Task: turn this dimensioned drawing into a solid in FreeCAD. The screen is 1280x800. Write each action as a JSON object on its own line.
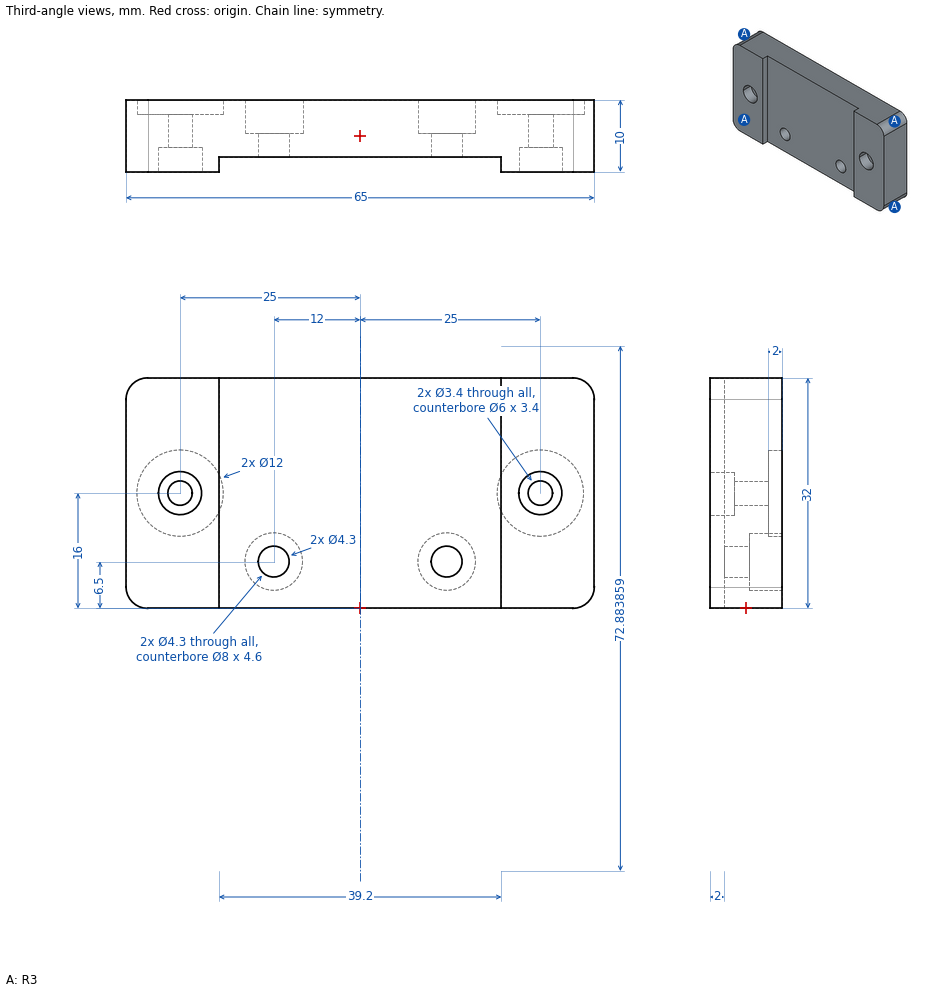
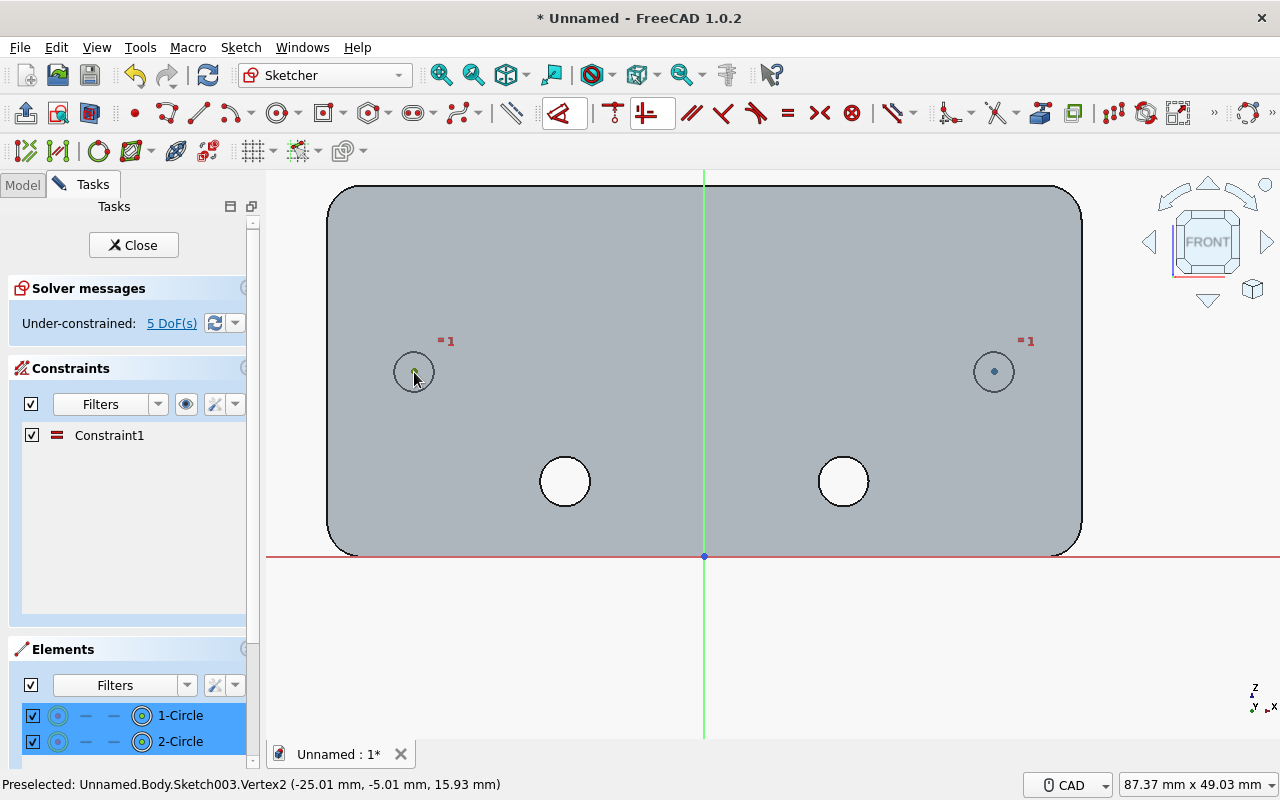
{"action": "left_click", "coordinate": [704, 674]}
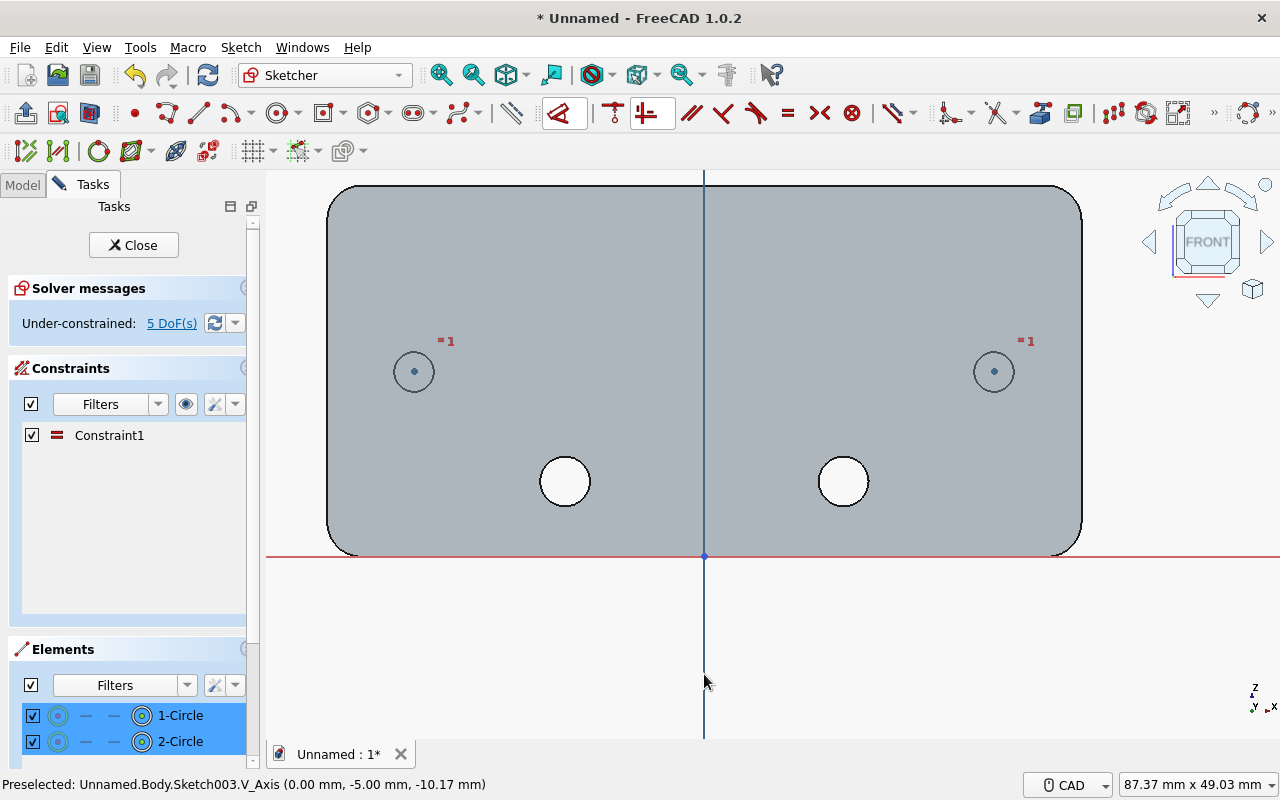
{"action": "left_click", "coordinate": [820, 114]}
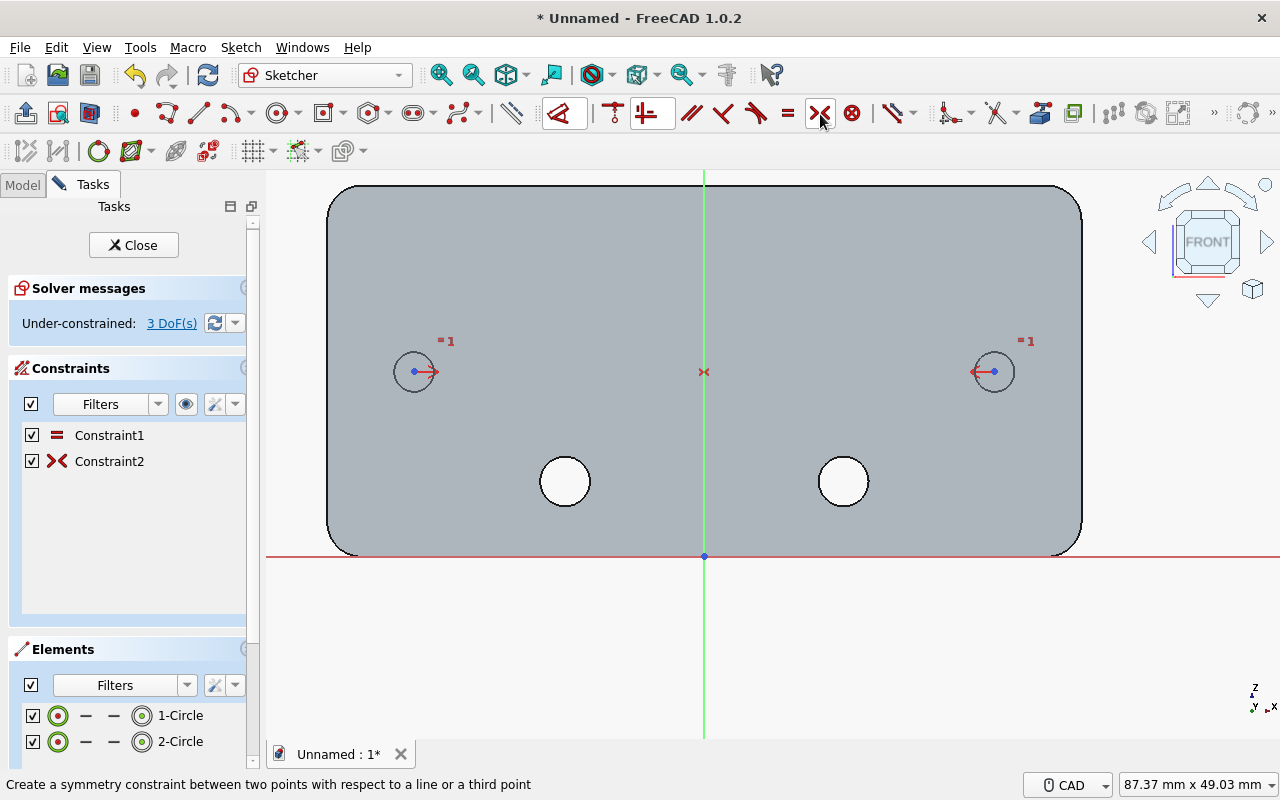
{"action": "left_click", "coordinate": [1009, 358]}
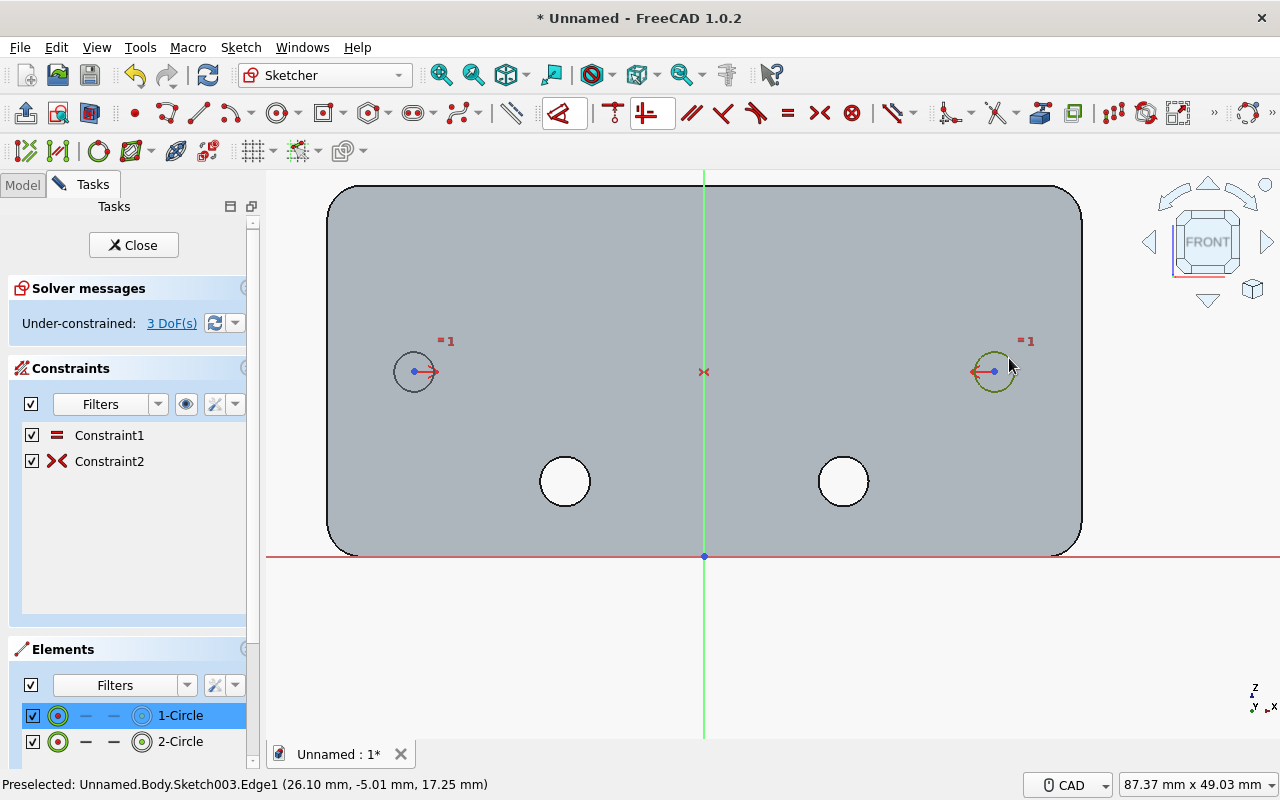
{"action": "key", "text": "k o"}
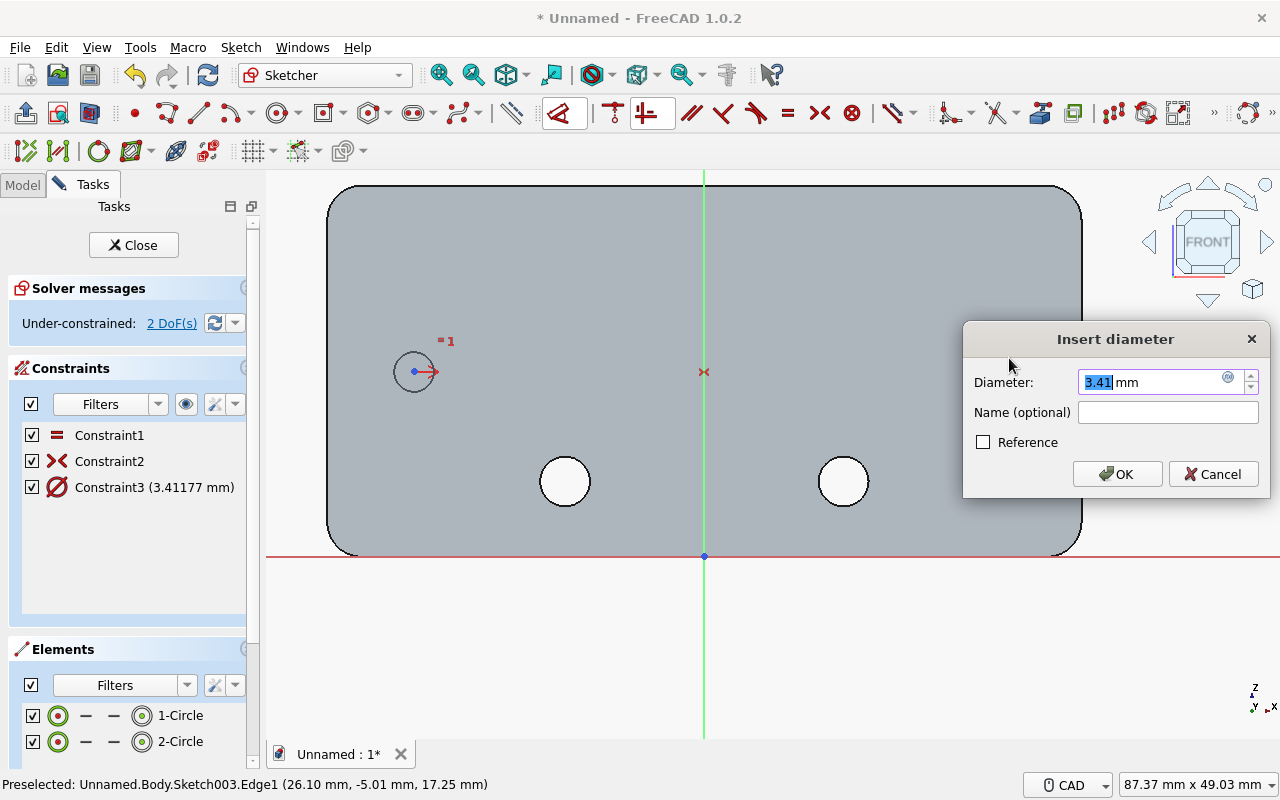
{"action": "type", "text": "3.4"}
{"action": "key", "text": "Return"}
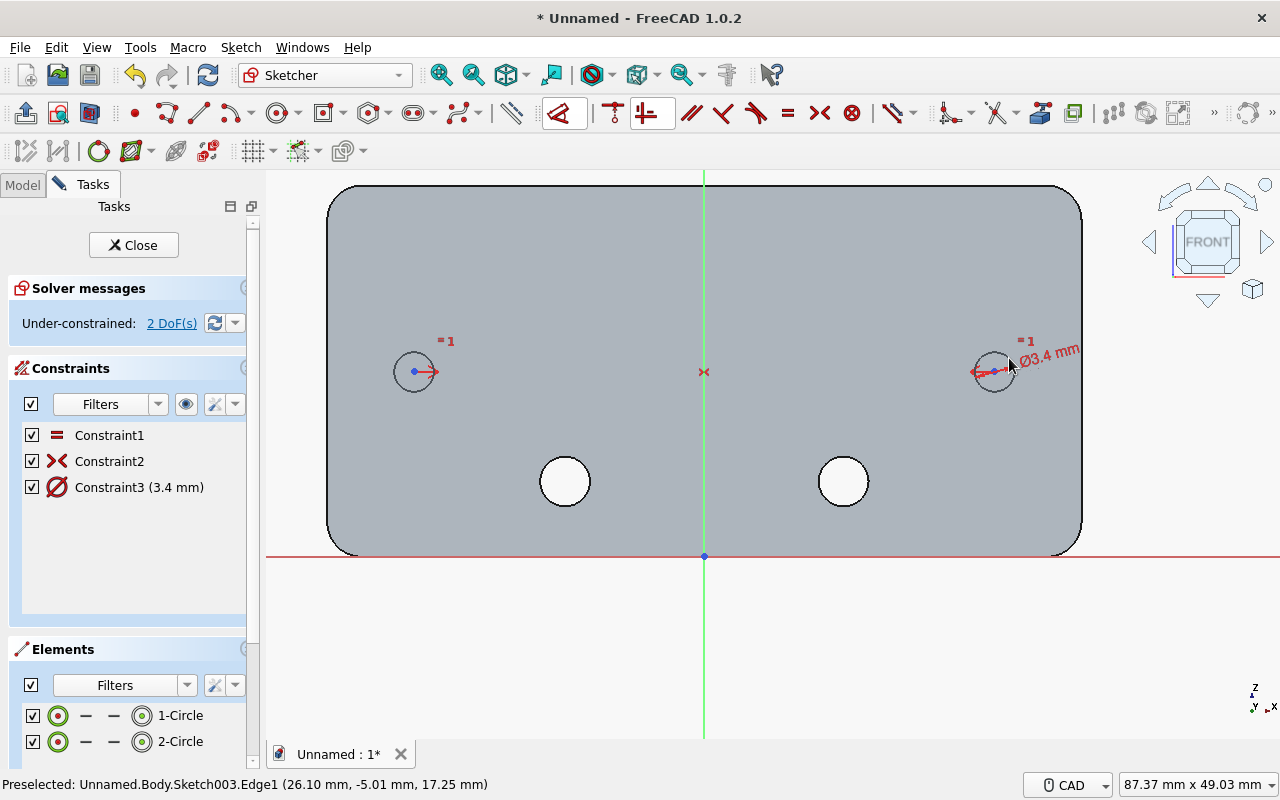
{"action": "left_click", "coordinate": [995, 372]}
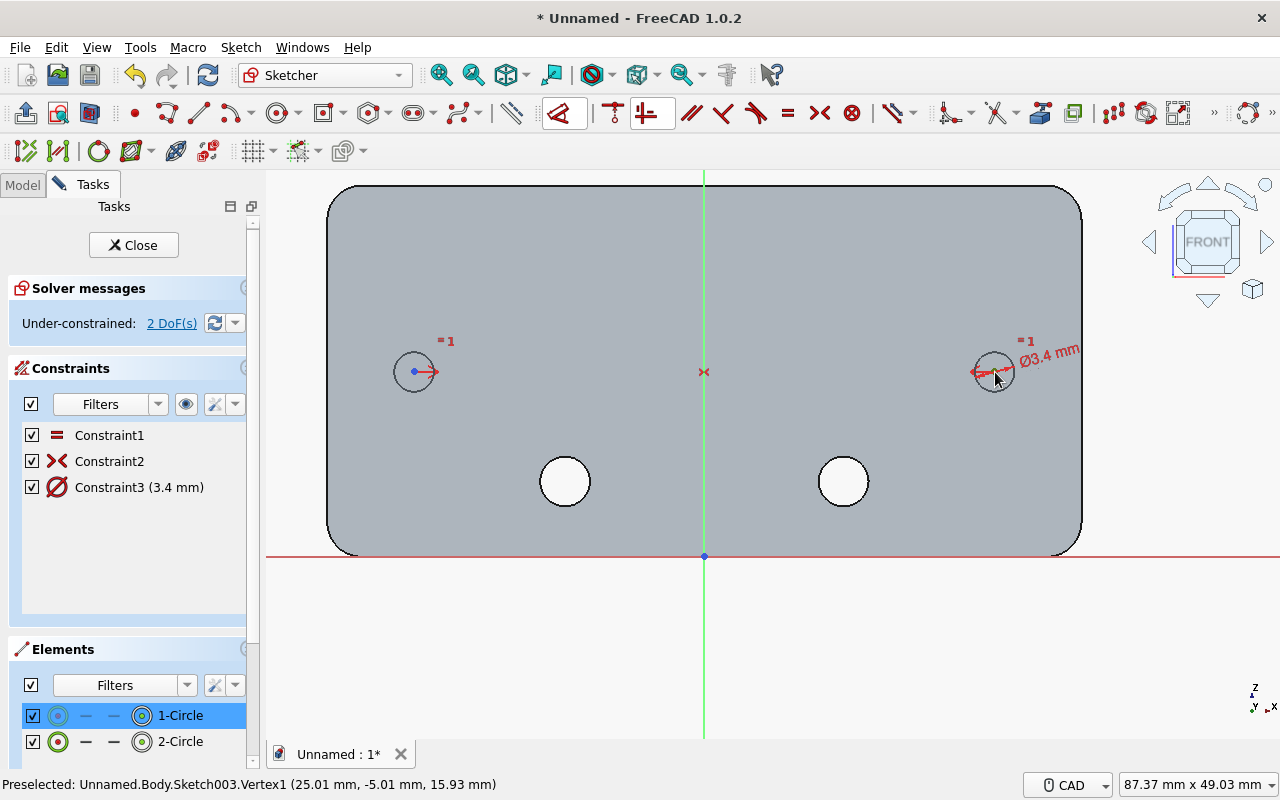
{"action": "left_click", "coordinate": [582, 114]}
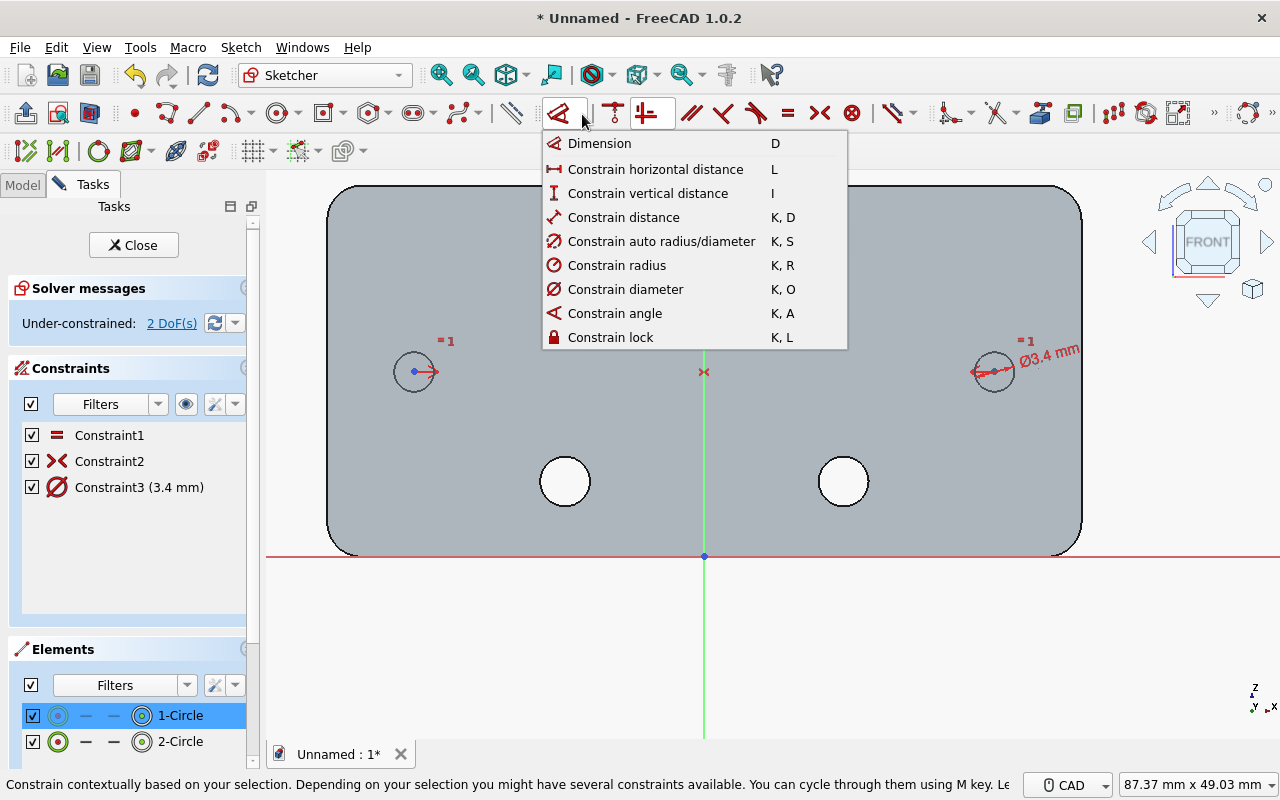
{"action": "left_click", "coordinate": [695, 169]}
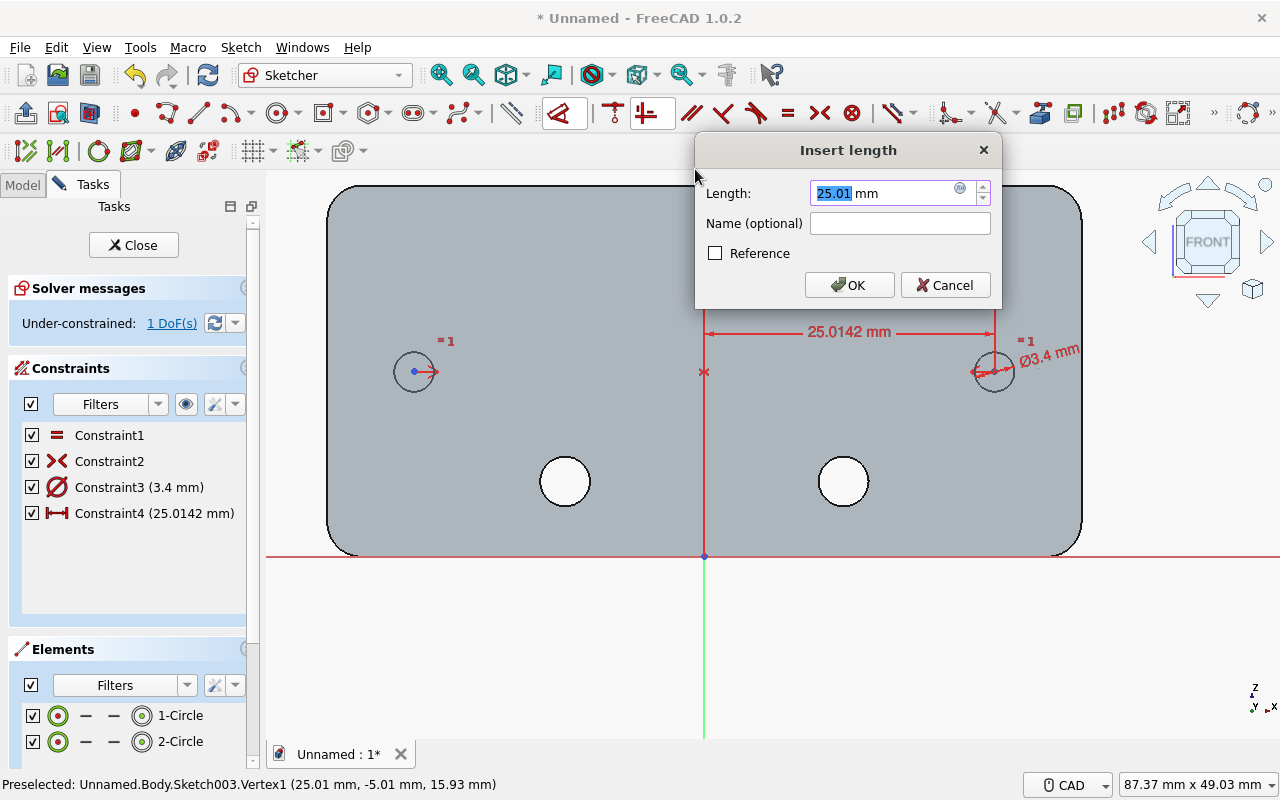
{"action": "type", "text": "25"}
{"action": "key", "text": "Return"}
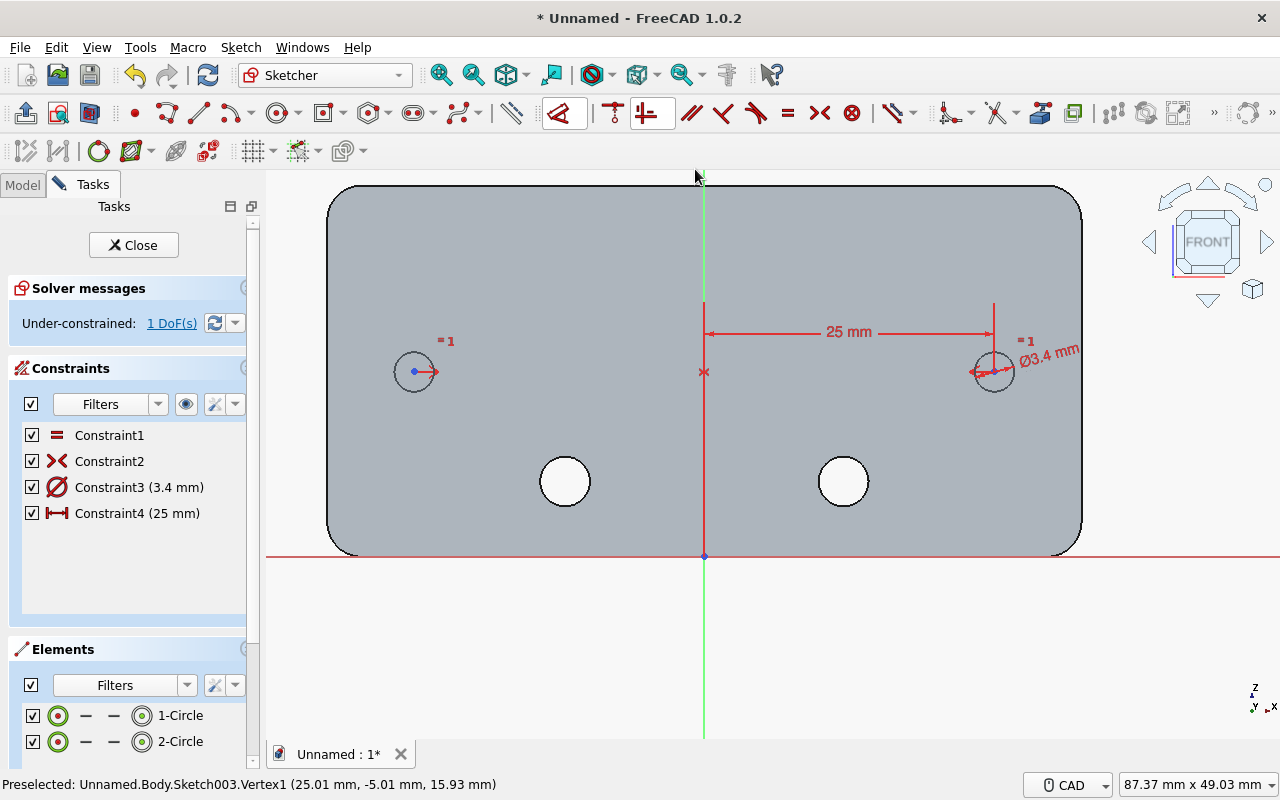
{"action": "left_click", "coordinate": [994, 372]}